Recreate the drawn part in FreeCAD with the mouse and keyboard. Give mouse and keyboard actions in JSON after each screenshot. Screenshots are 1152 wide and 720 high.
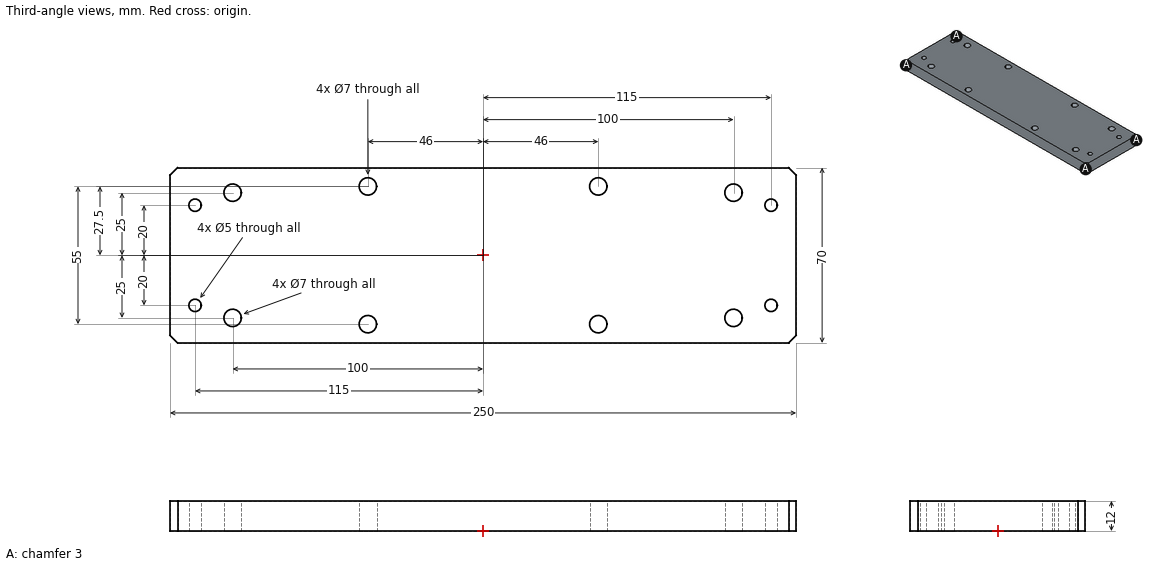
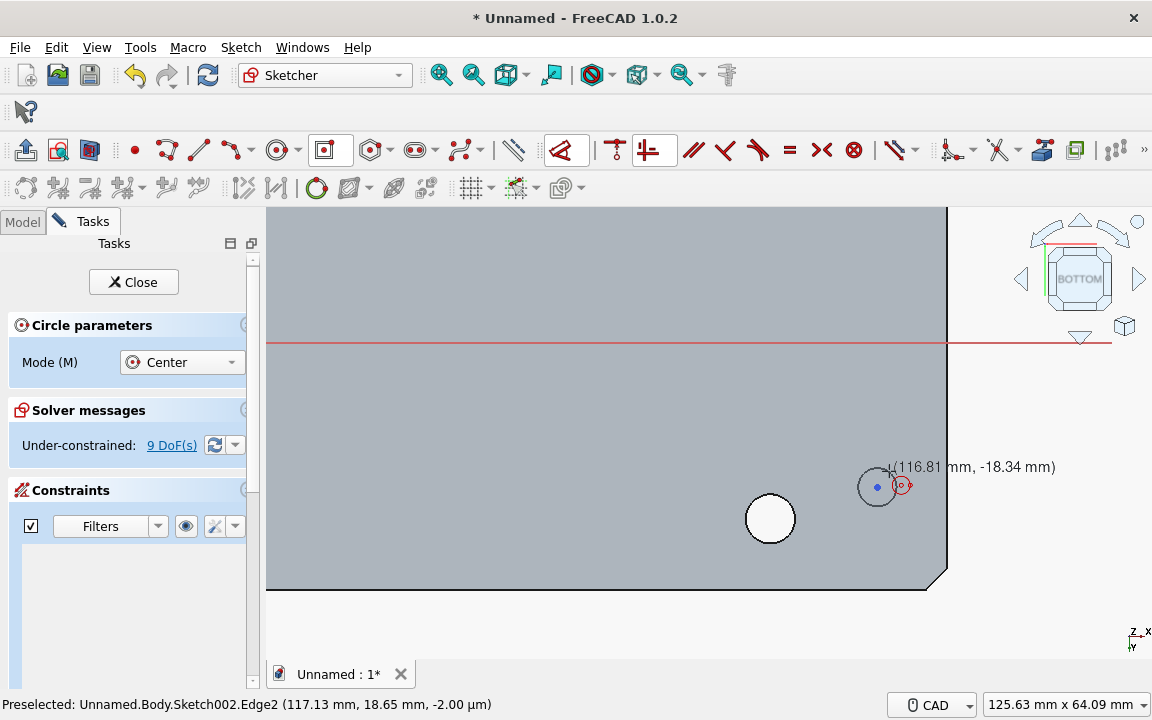
{"action": "scroll", "coordinate": [888, 472], "scroll_direction": "down", "scroll_amount": 6}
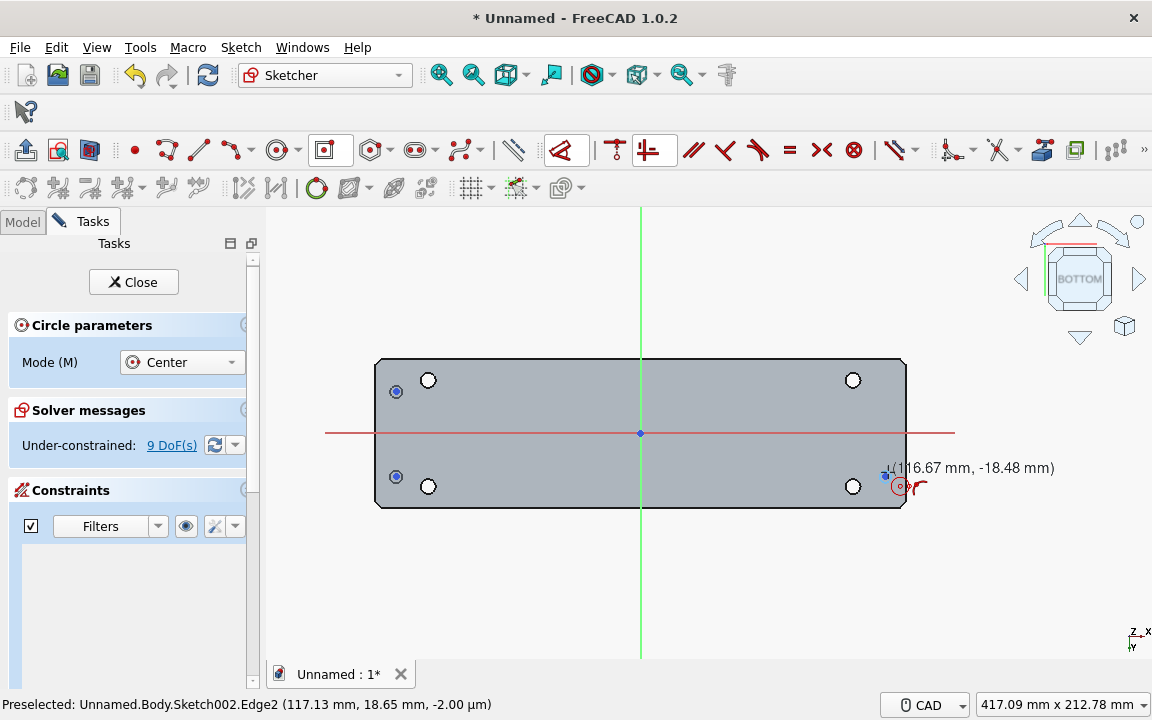
{"action": "scroll", "coordinate": [885, 391], "scroll_direction": "up", "scroll_amount": 8}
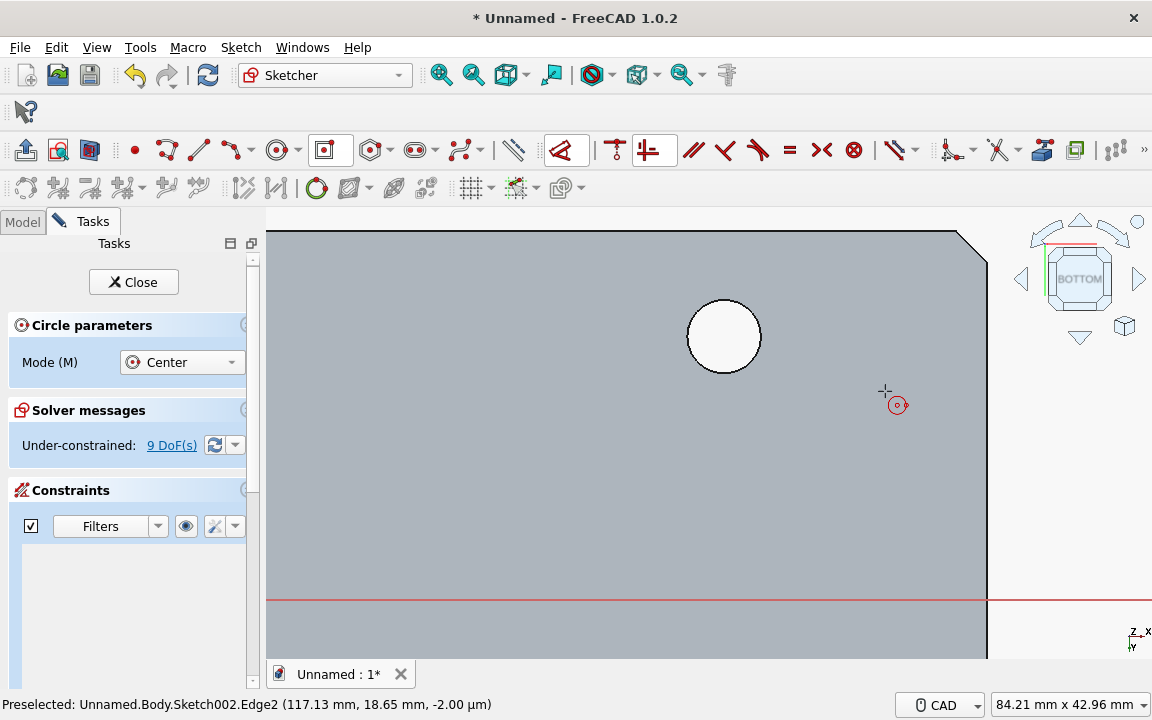
{"action": "scroll", "coordinate": [885, 391], "scroll_direction": "down", "scroll_amount": 8}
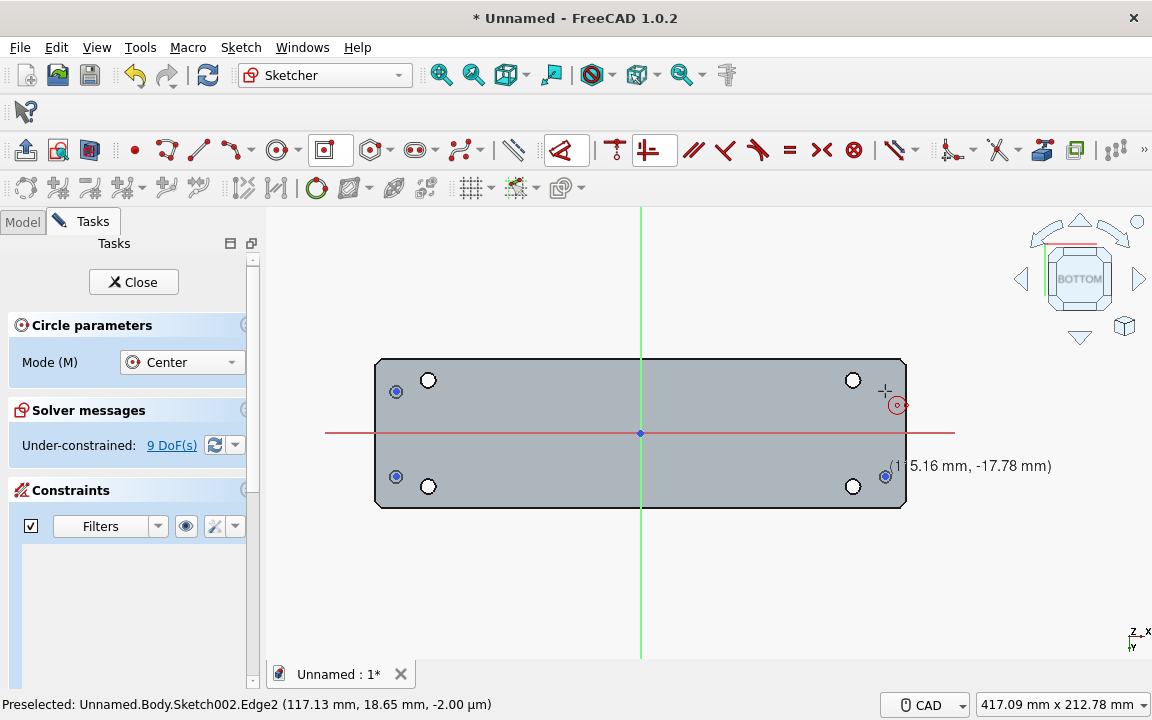
{"action": "left_click", "coordinate": [885, 391]}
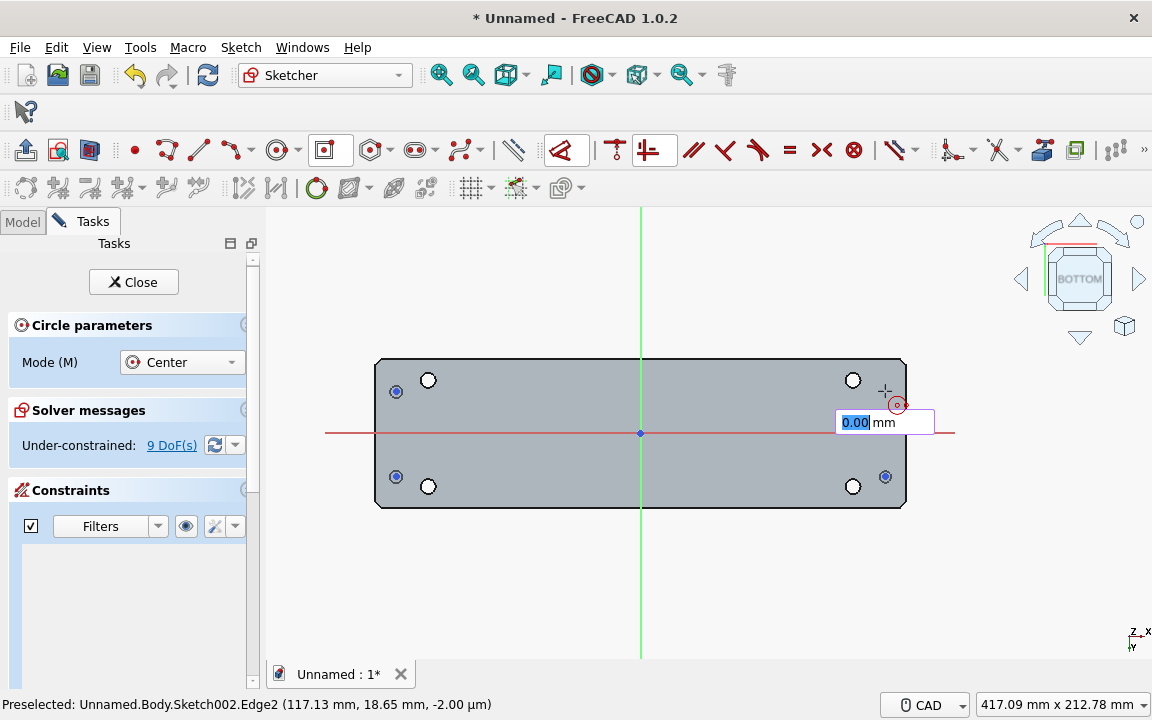
{"action": "scroll", "coordinate": [889, 387], "scroll_direction": "up", "scroll_amount": 6}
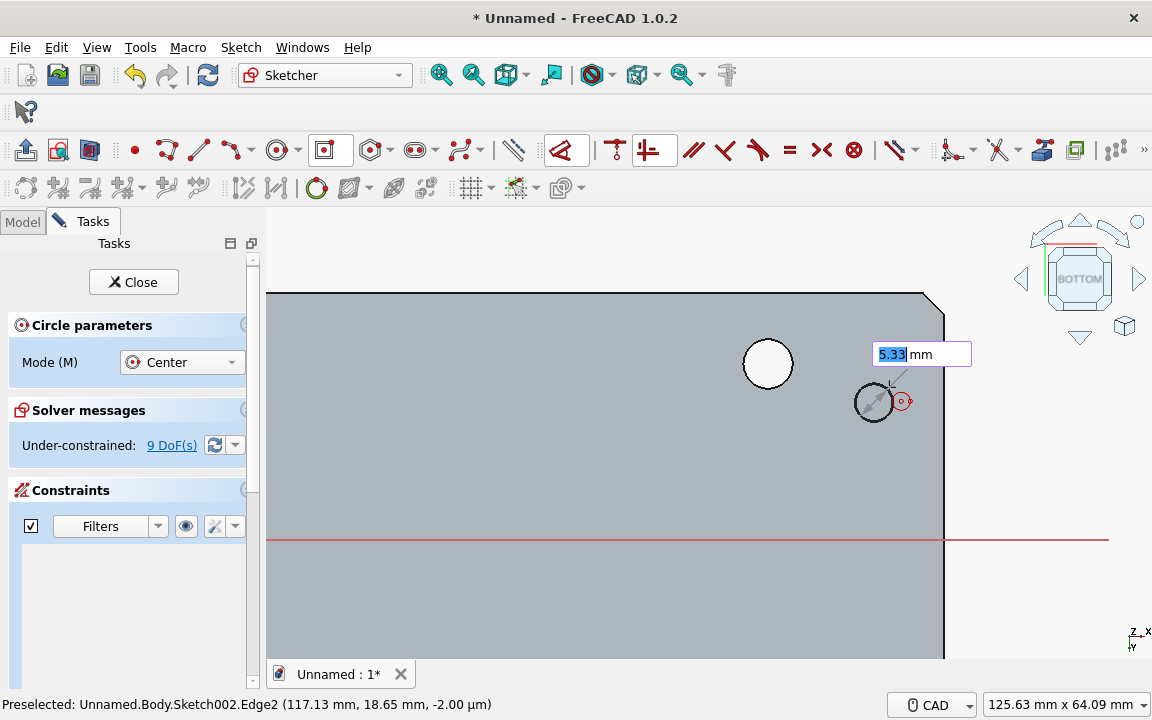
{"action": "left_click", "coordinate": [886, 387]}
{"action": "key", "text": "Escape"}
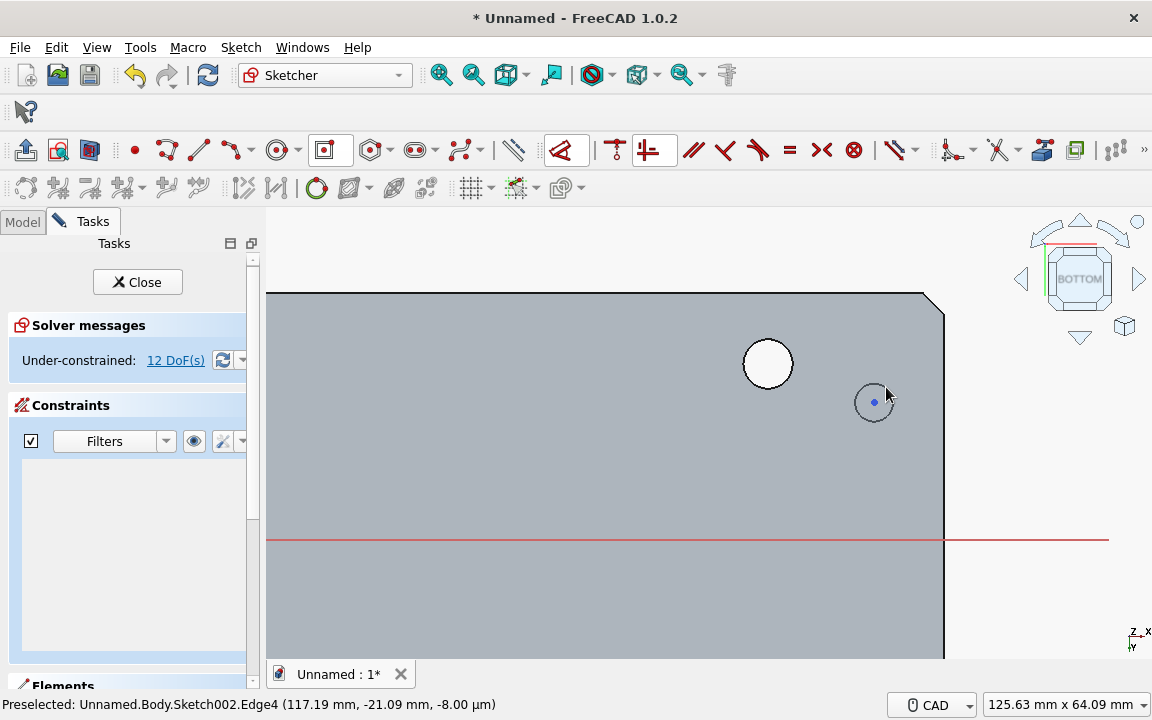
{"action": "scroll", "coordinate": [889, 387], "scroll_direction": "down", "scroll_amount": 6}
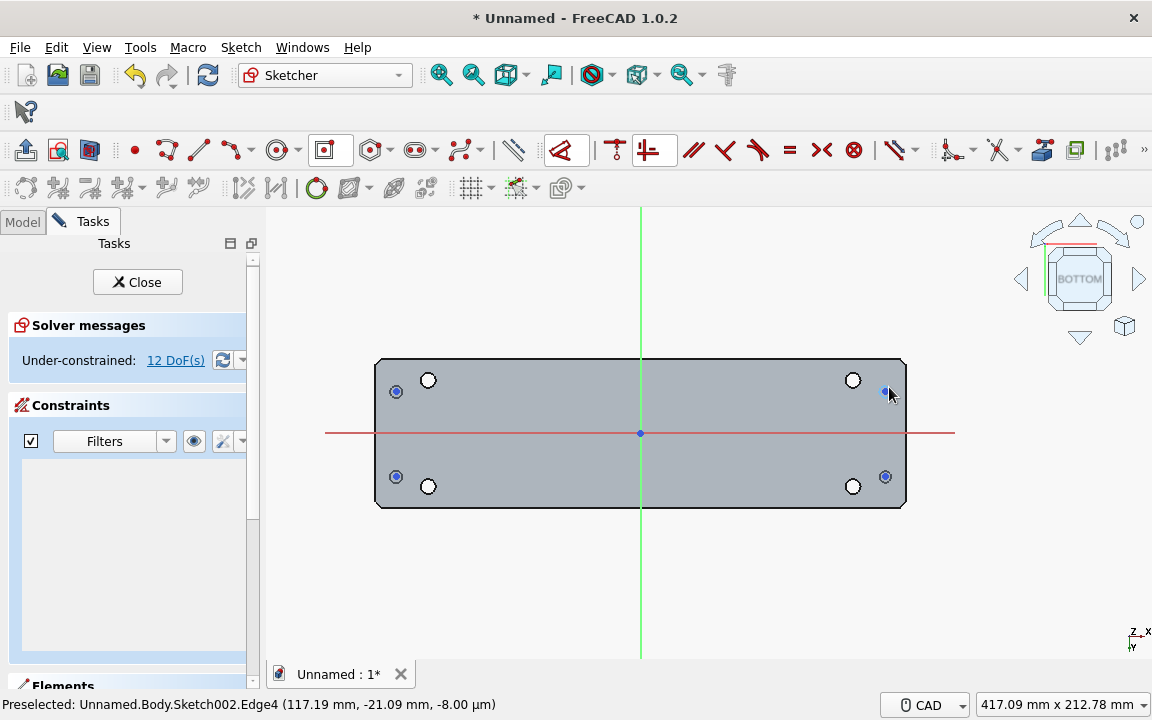
{"action": "scroll", "coordinate": [400, 388], "scroll_direction": "up", "scroll_amount": 5}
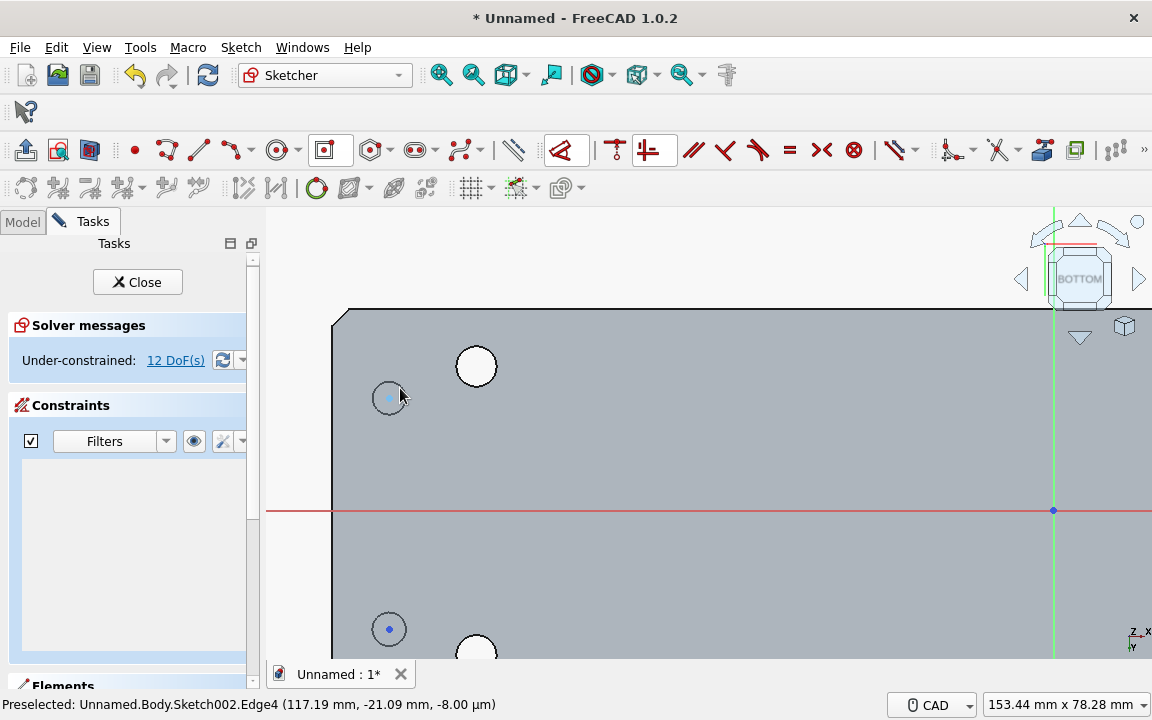
{"action": "left_click", "coordinate": [401, 387]}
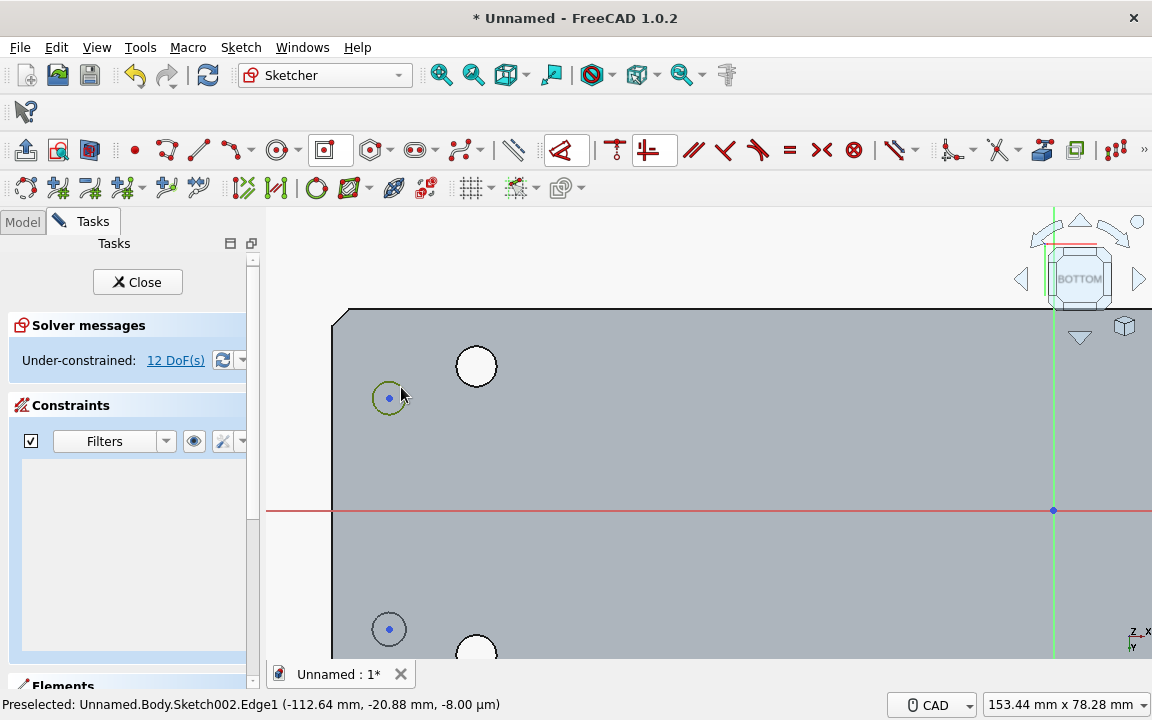
{"action": "left_click", "coordinate": [401, 617]}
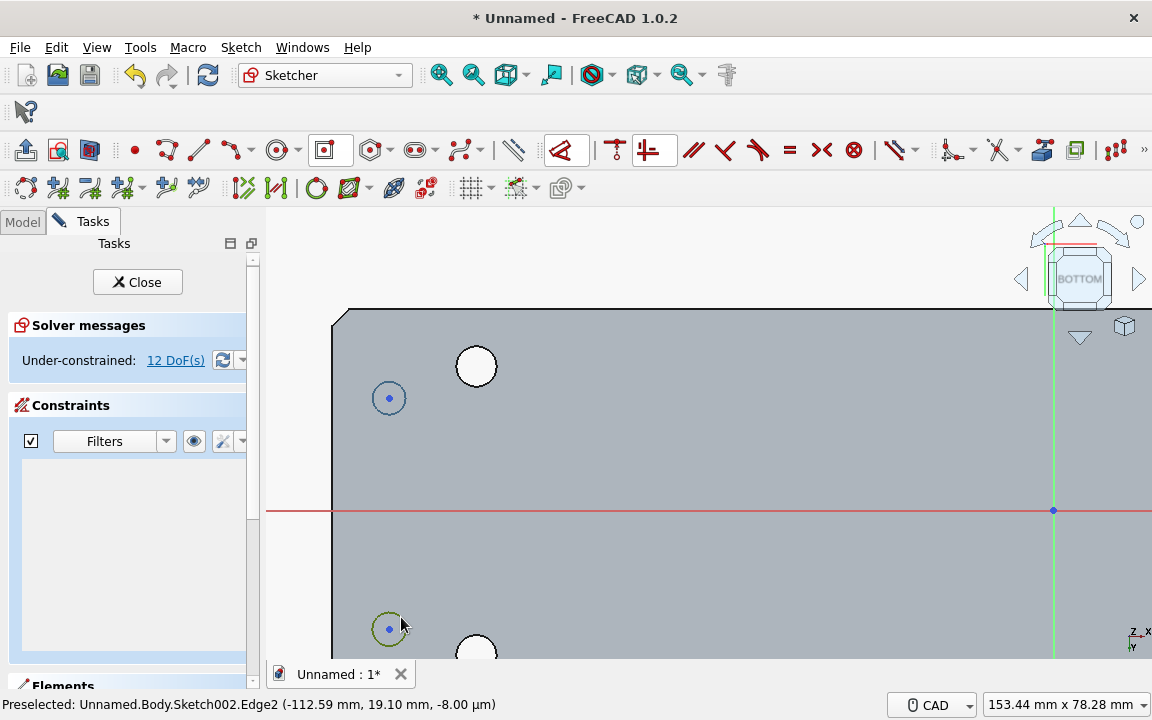
{"action": "scroll", "coordinate": [400, 388], "scroll_direction": "down", "scroll_amount": 5}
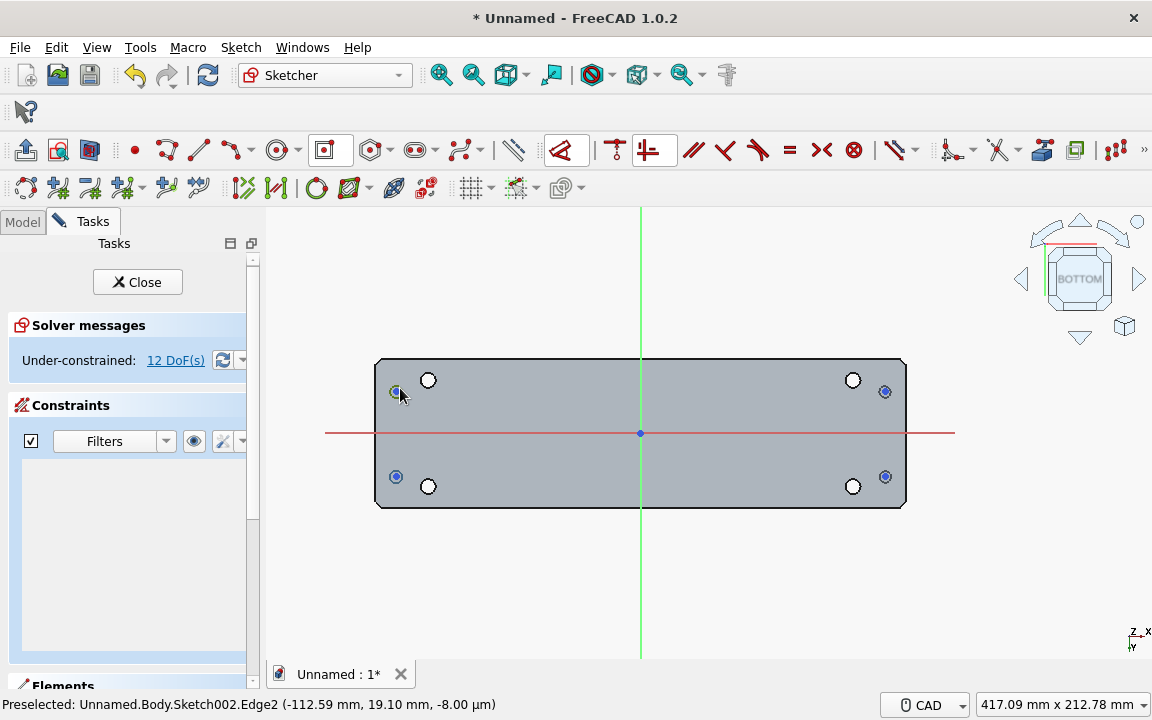
{"action": "scroll", "coordinate": [889, 473], "scroll_direction": "up", "scroll_amount": 5}